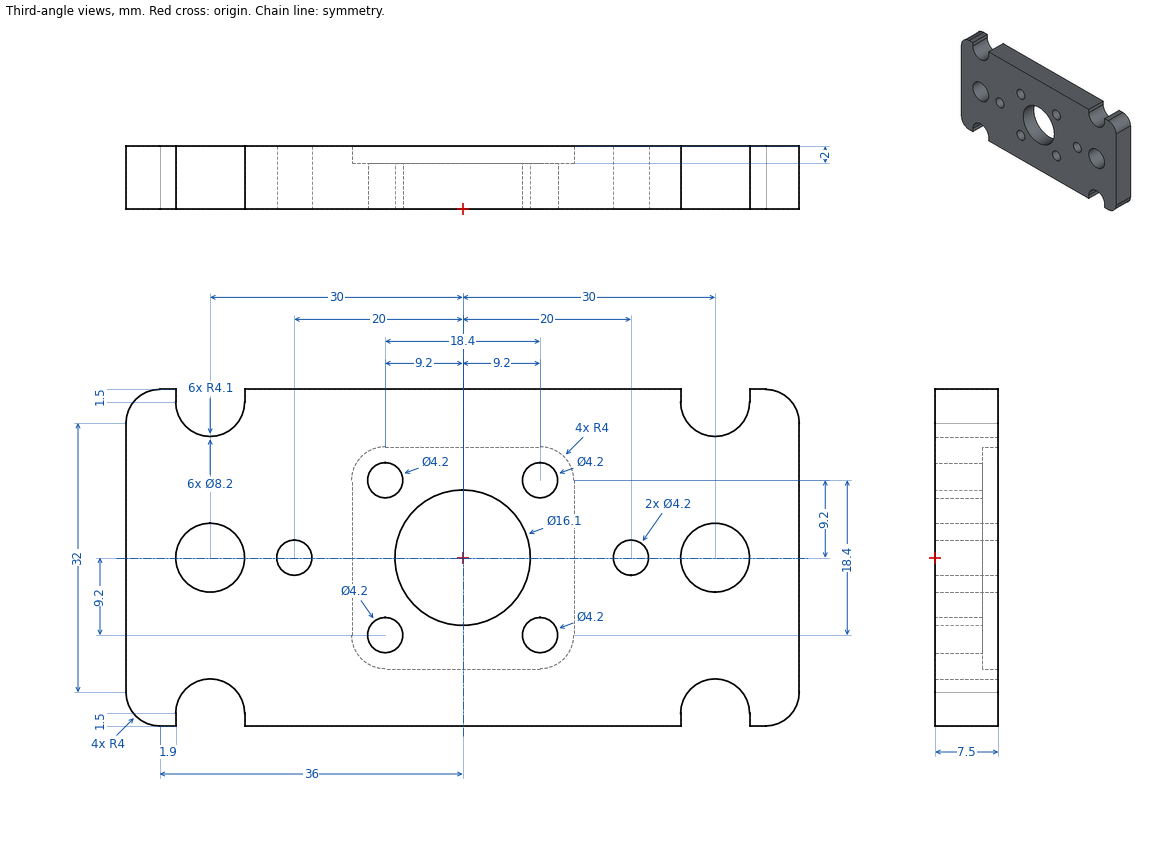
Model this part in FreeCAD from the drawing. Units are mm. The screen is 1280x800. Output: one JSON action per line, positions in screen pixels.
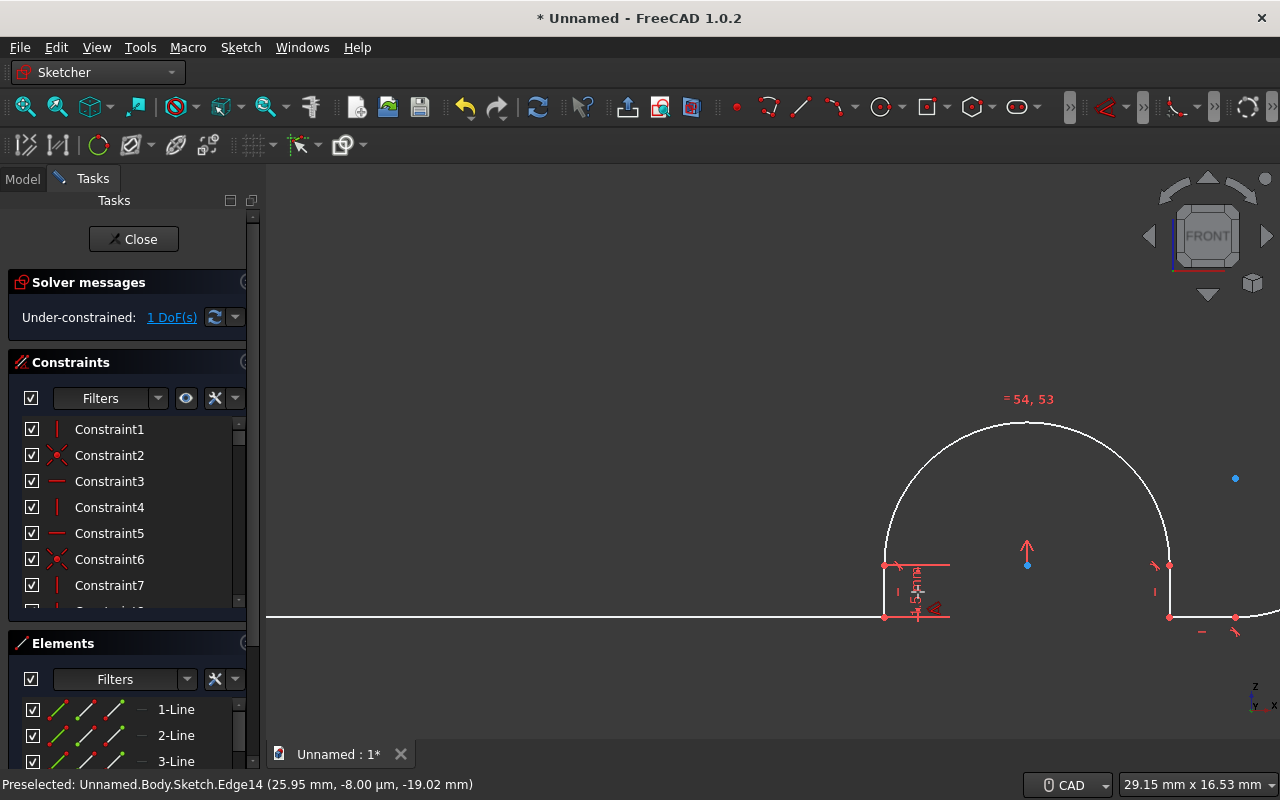
{"action": "scroll", "coordinate": [887, 586], "scroll_direction": "down", "scroll_amount": 8}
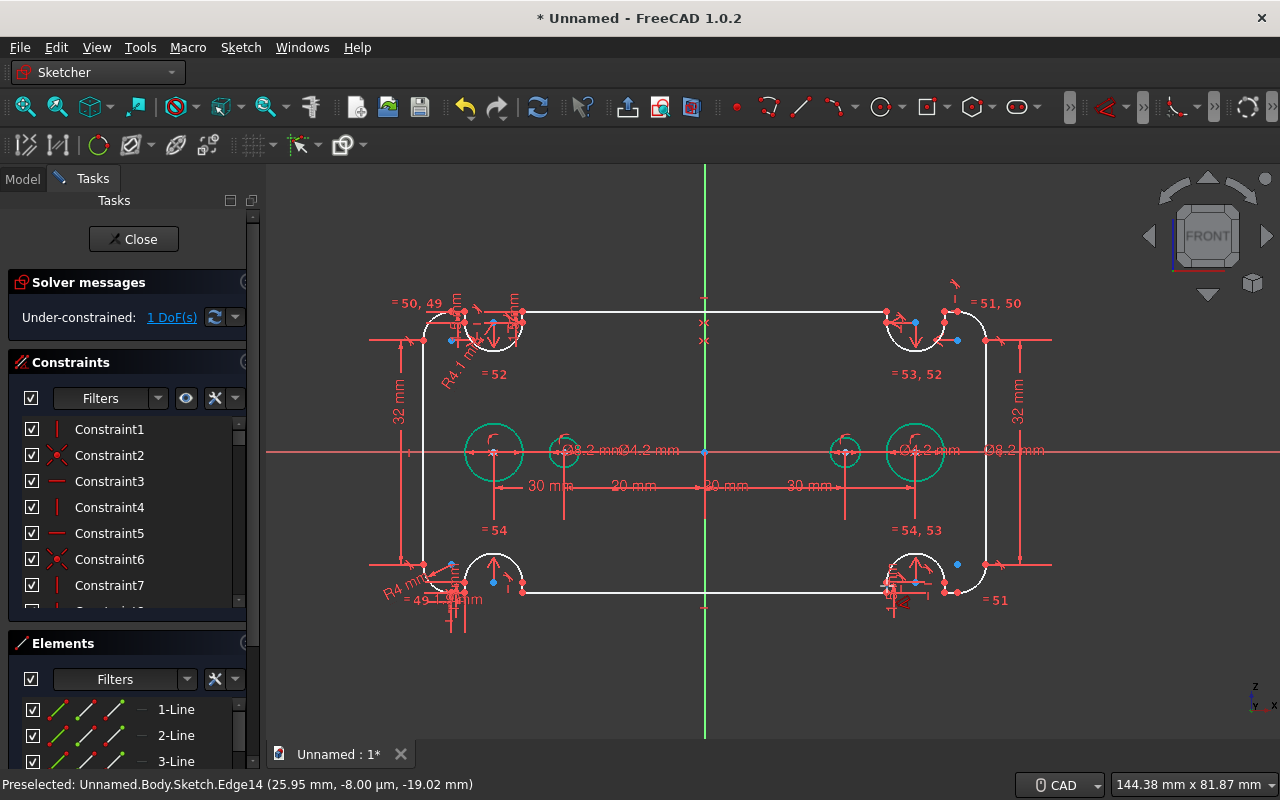
{"action": "left_click", "coordinate": [451, 593]}
{"action": "left_click", "coordinate": [578, 627]}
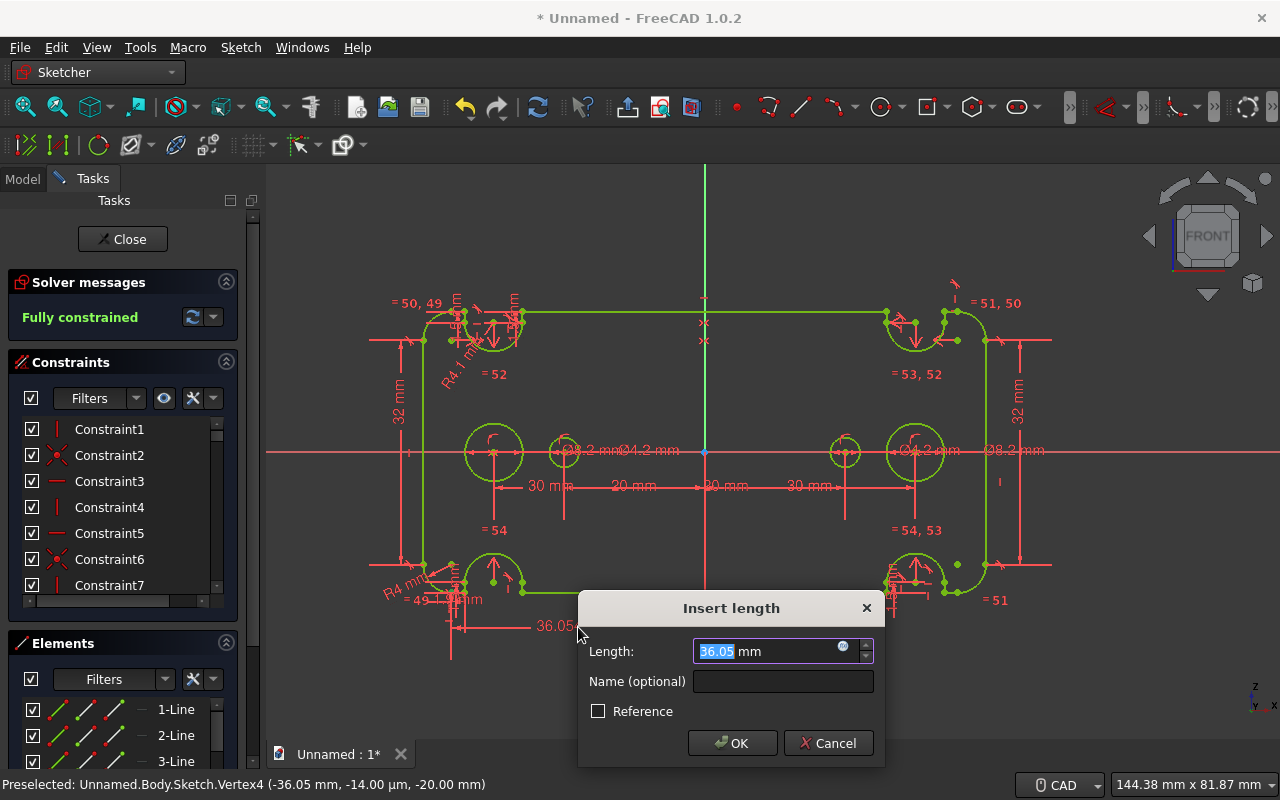
{"action": "type", "text": "36"}
{"action": "key", "text": "Return"}
{"action": "key", "text": "Escape"}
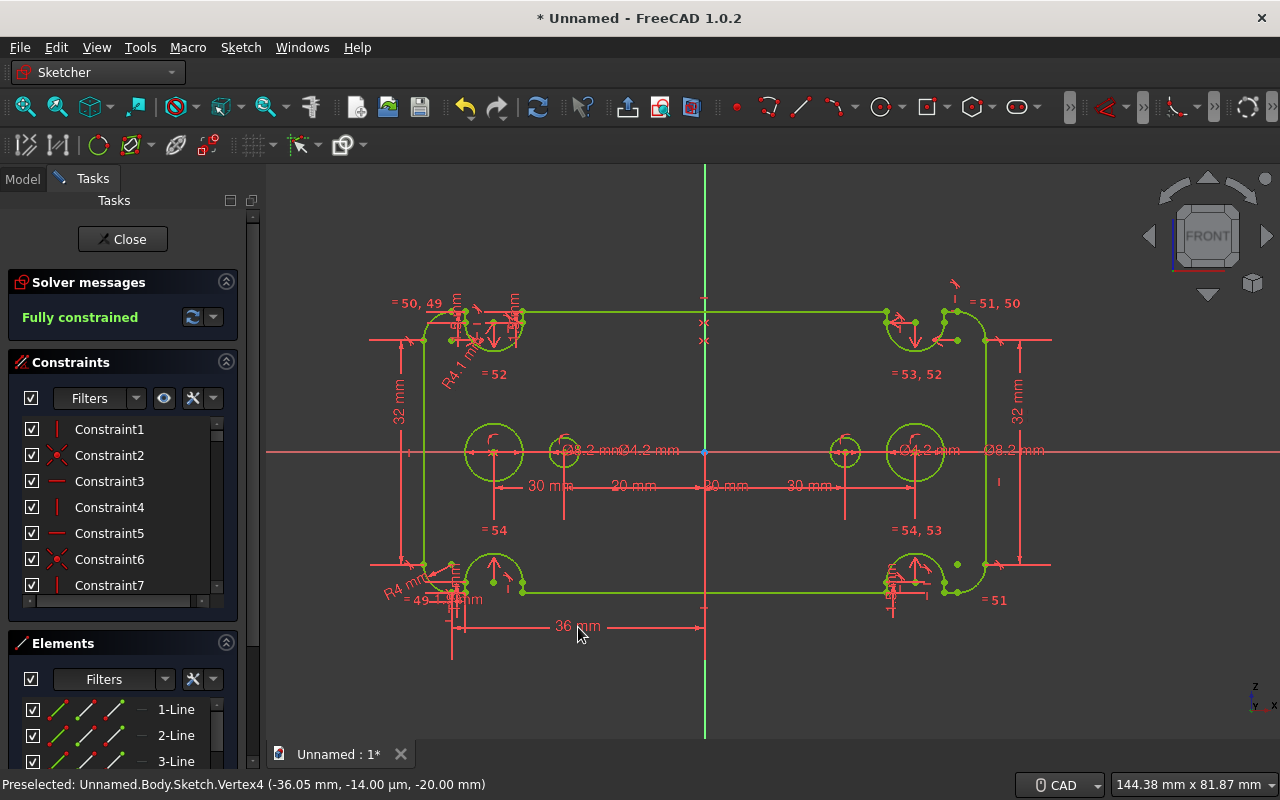
{"action": "left_click", "coordinate": [123, 239]}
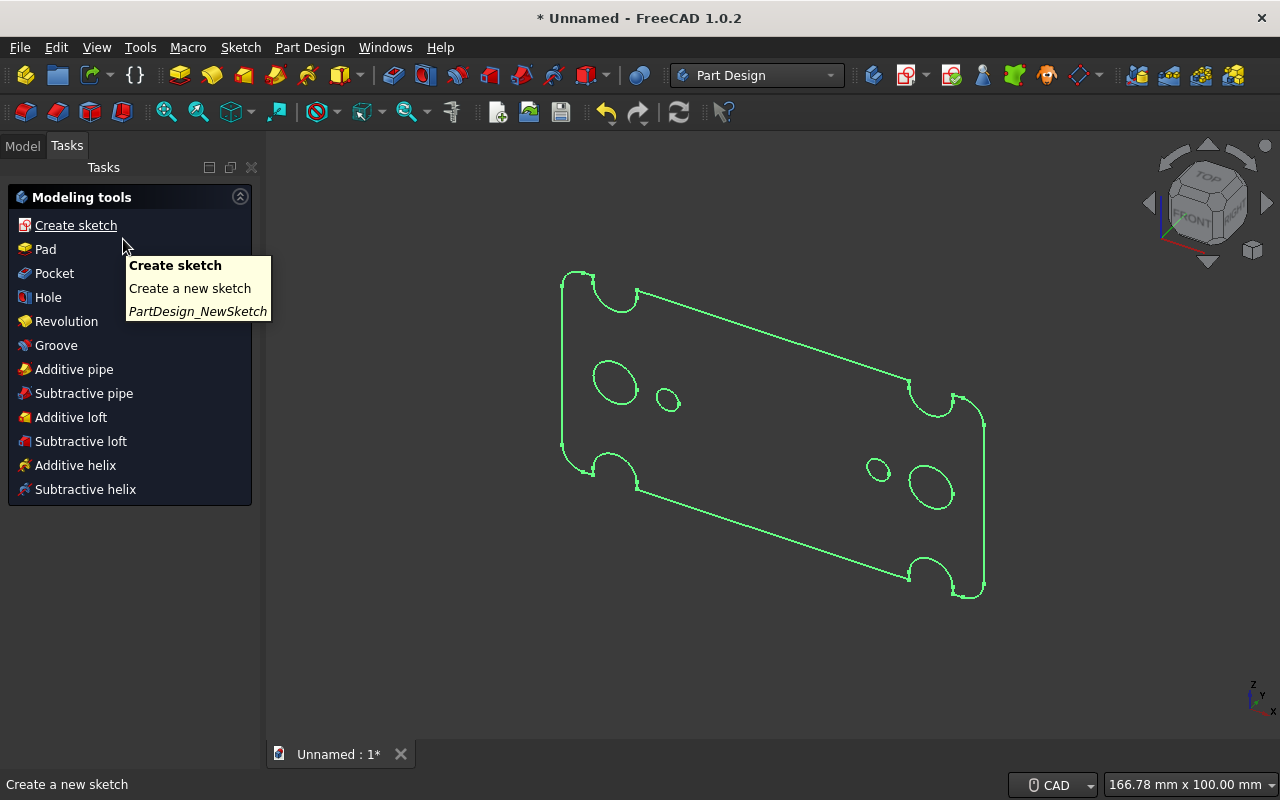
{"action": "left_click", "coordinate": [180, 76]}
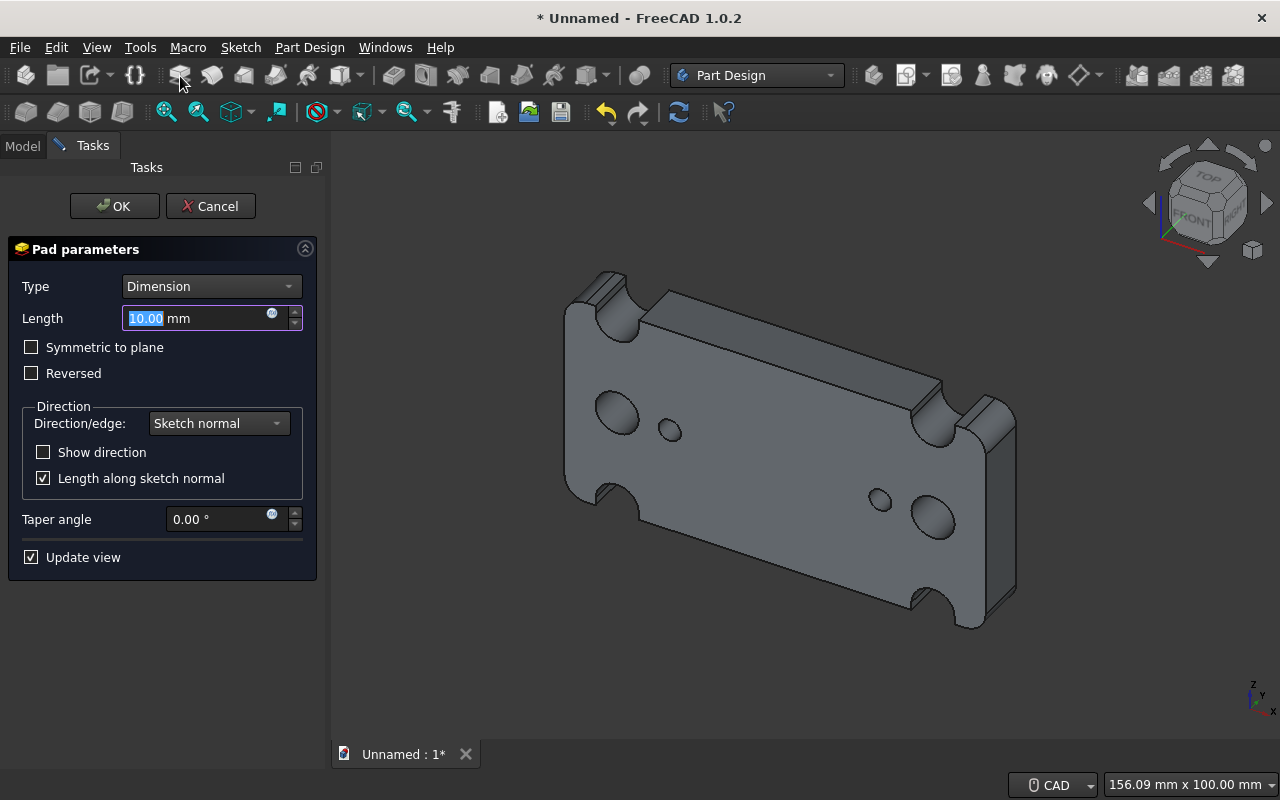
{"action": "type", "text": "7.5"}
{"action": "key", "text": "Tab"}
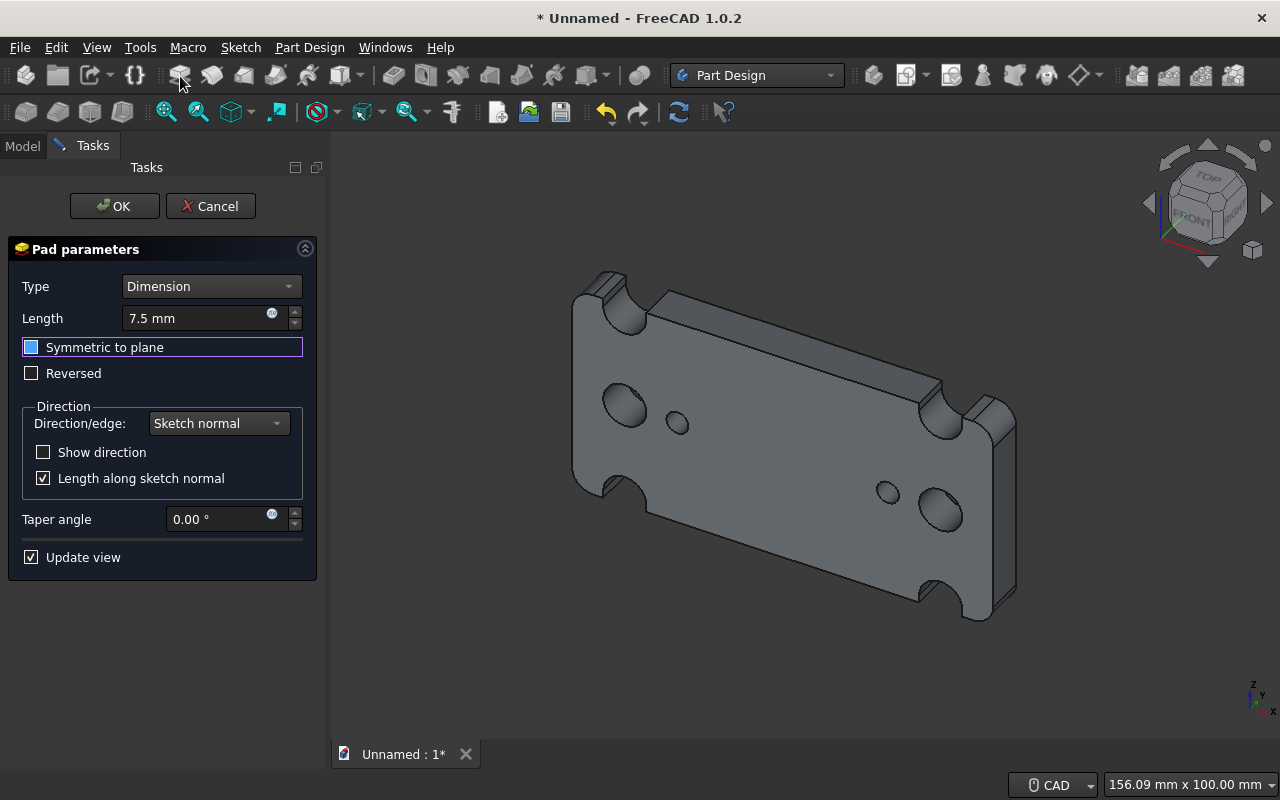
{"action": "left_click", "coordinate": [30, 373]}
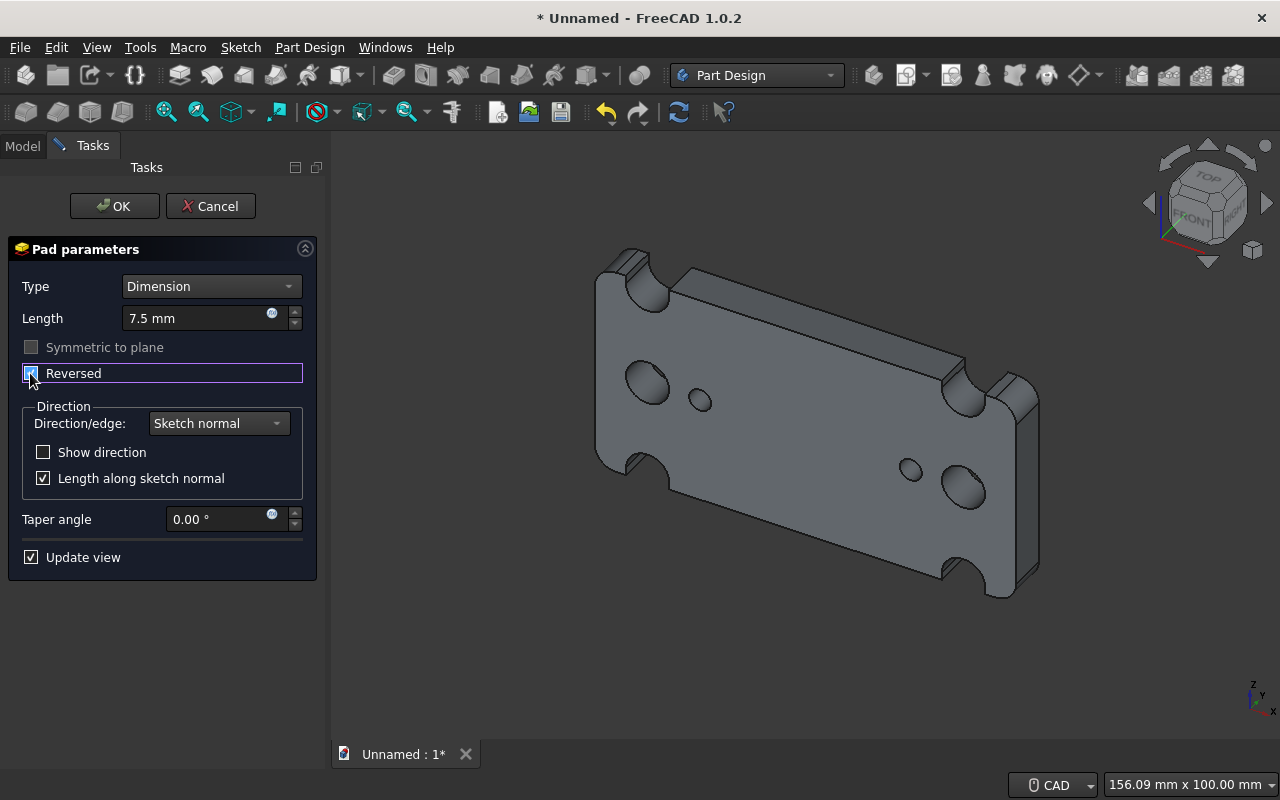
{"action": "left_click", "coordinate": [115, 206]}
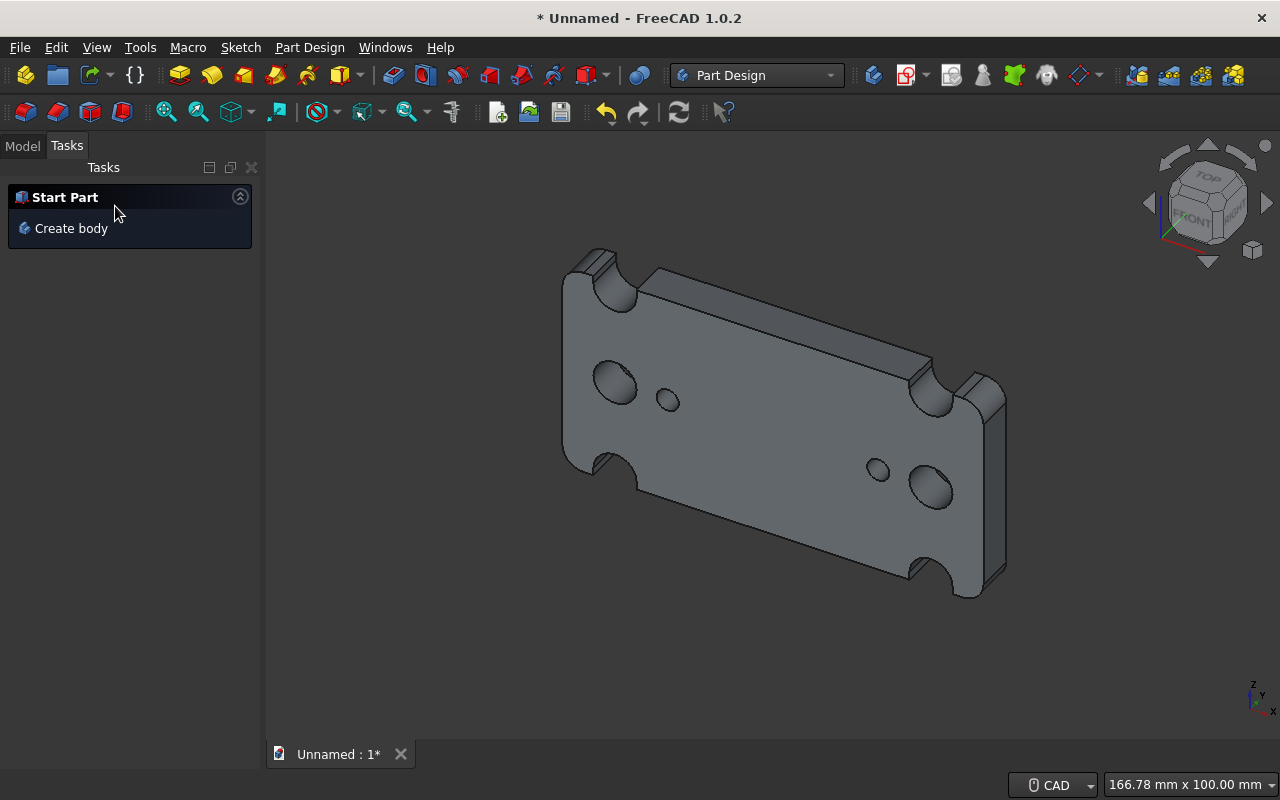
{"action": "key", "text": "4"}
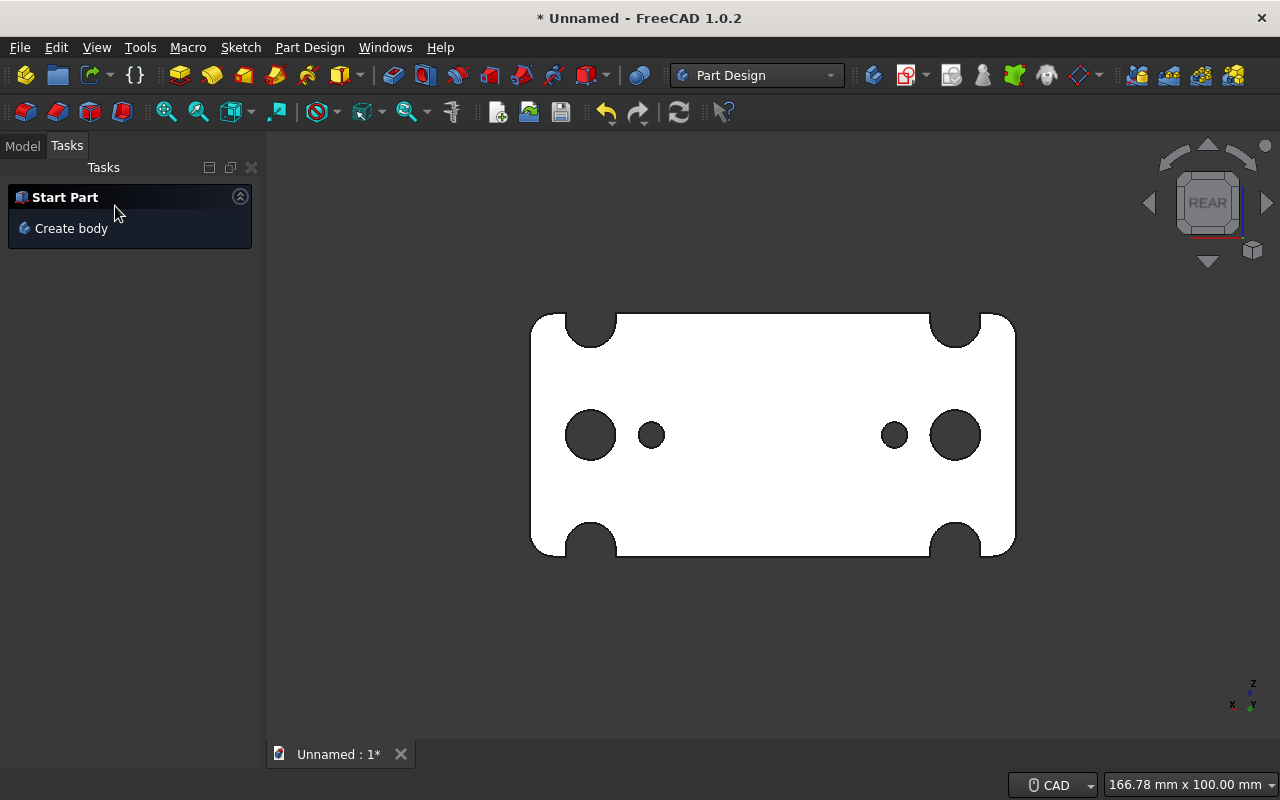
{"action": "left_click", "coordinate": [773, 434]}